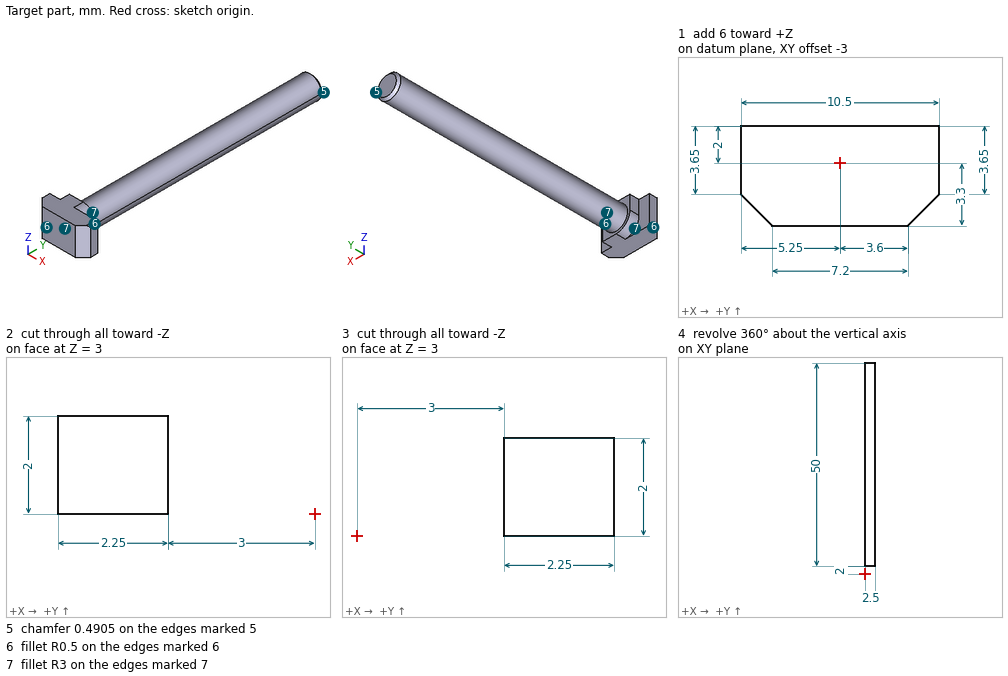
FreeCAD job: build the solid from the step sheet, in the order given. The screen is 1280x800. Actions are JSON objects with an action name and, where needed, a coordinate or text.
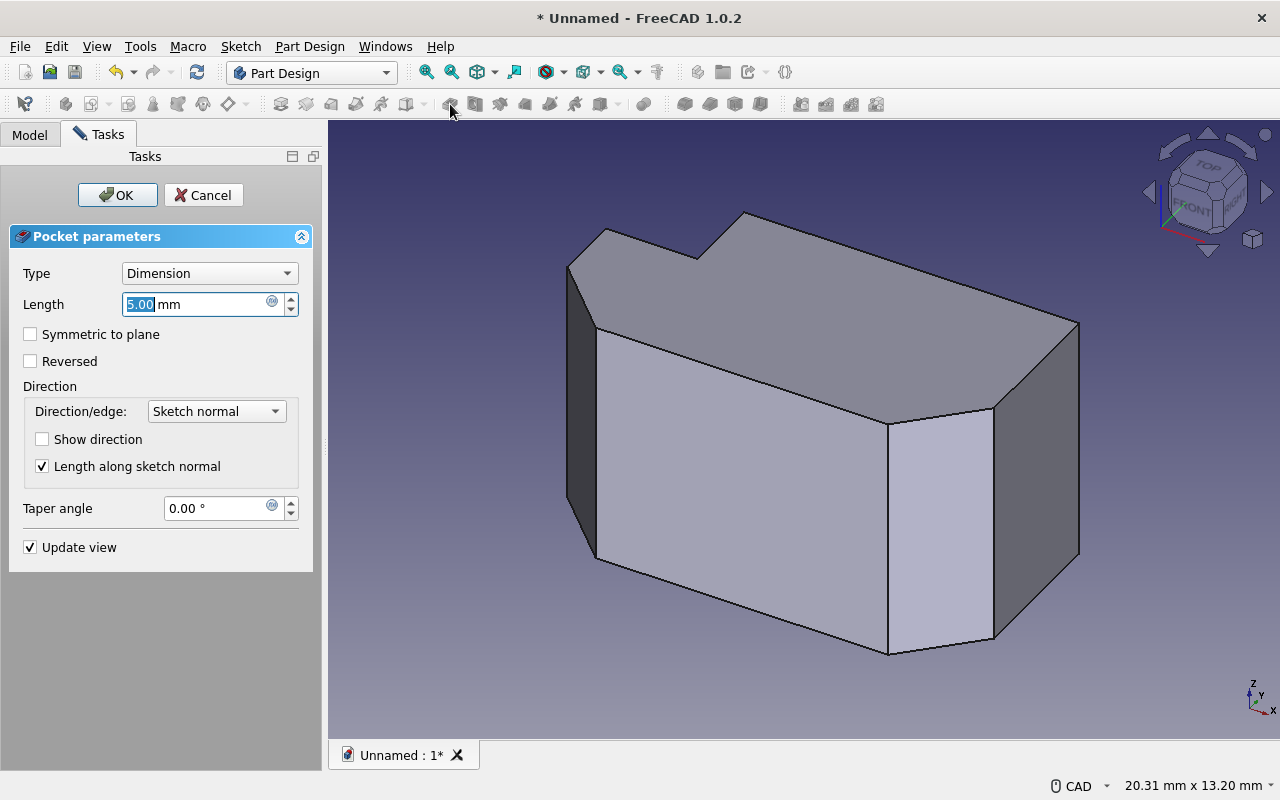
{"action": "left_click", "coordinate": [210, 274]}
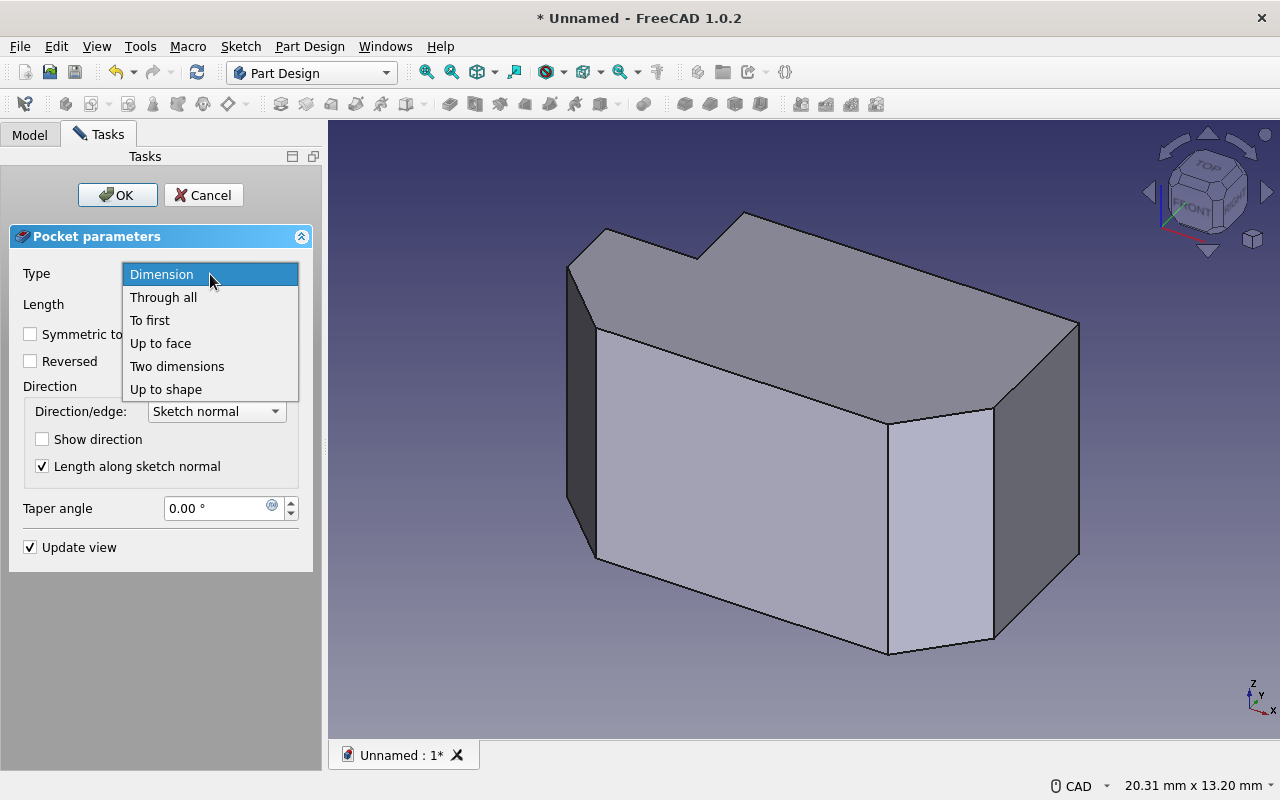
{"action": "left_click", "coordinate": [208, 298]}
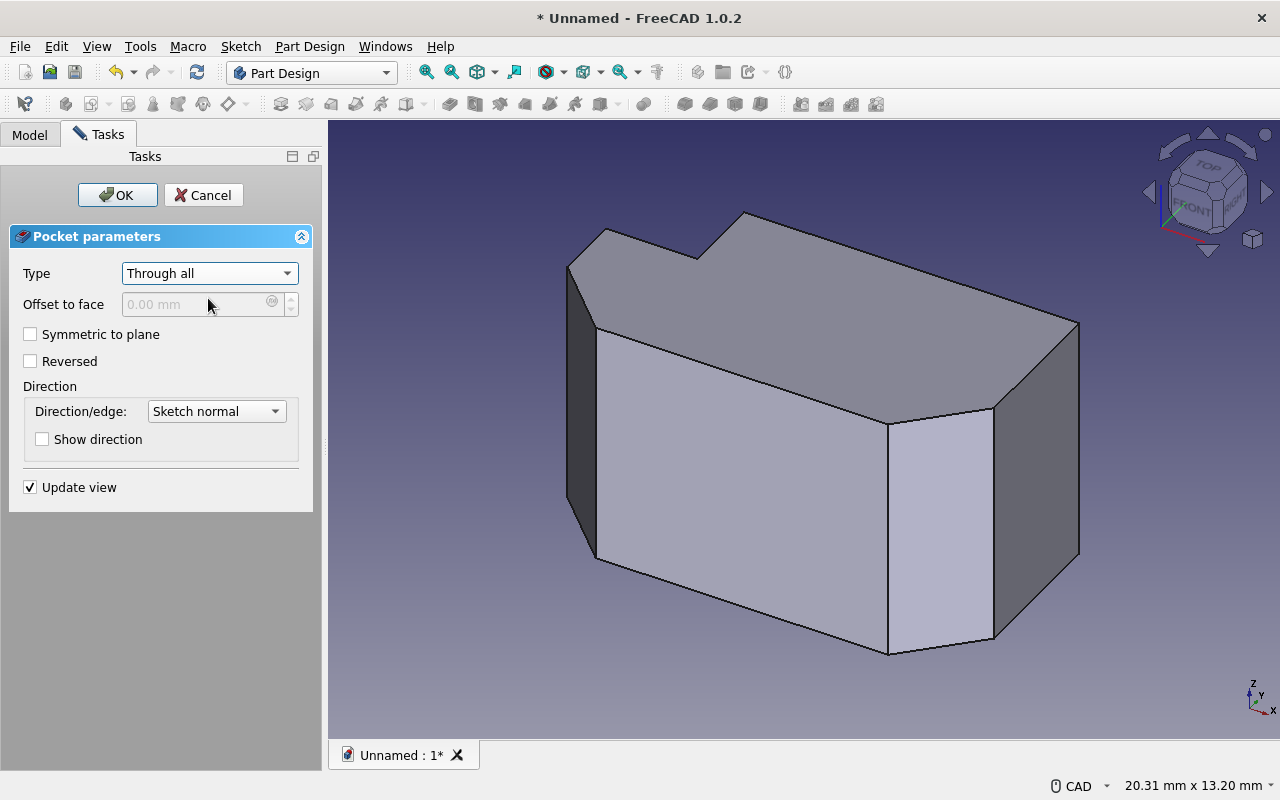
{"action": "left_click", "coordinate": [118, 195]}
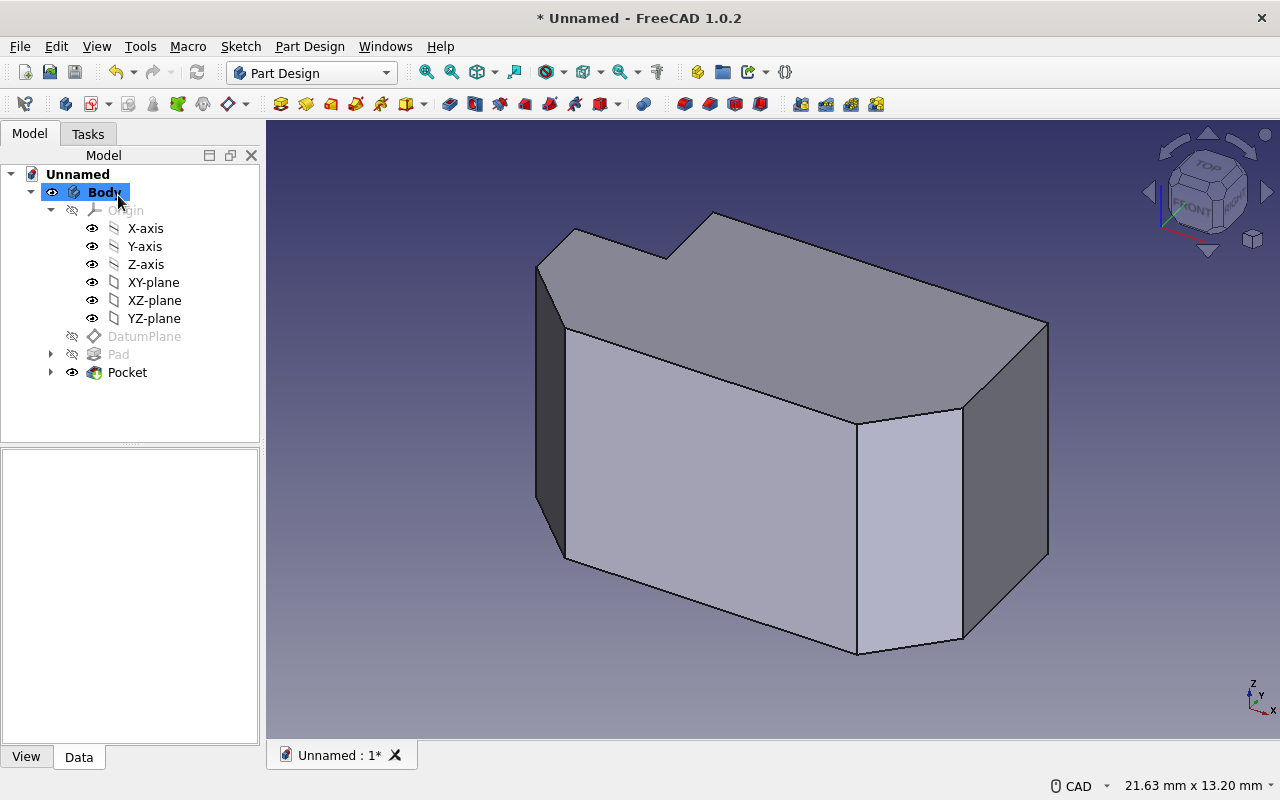
{"action": "left_click", "coordinate": [834, 333]}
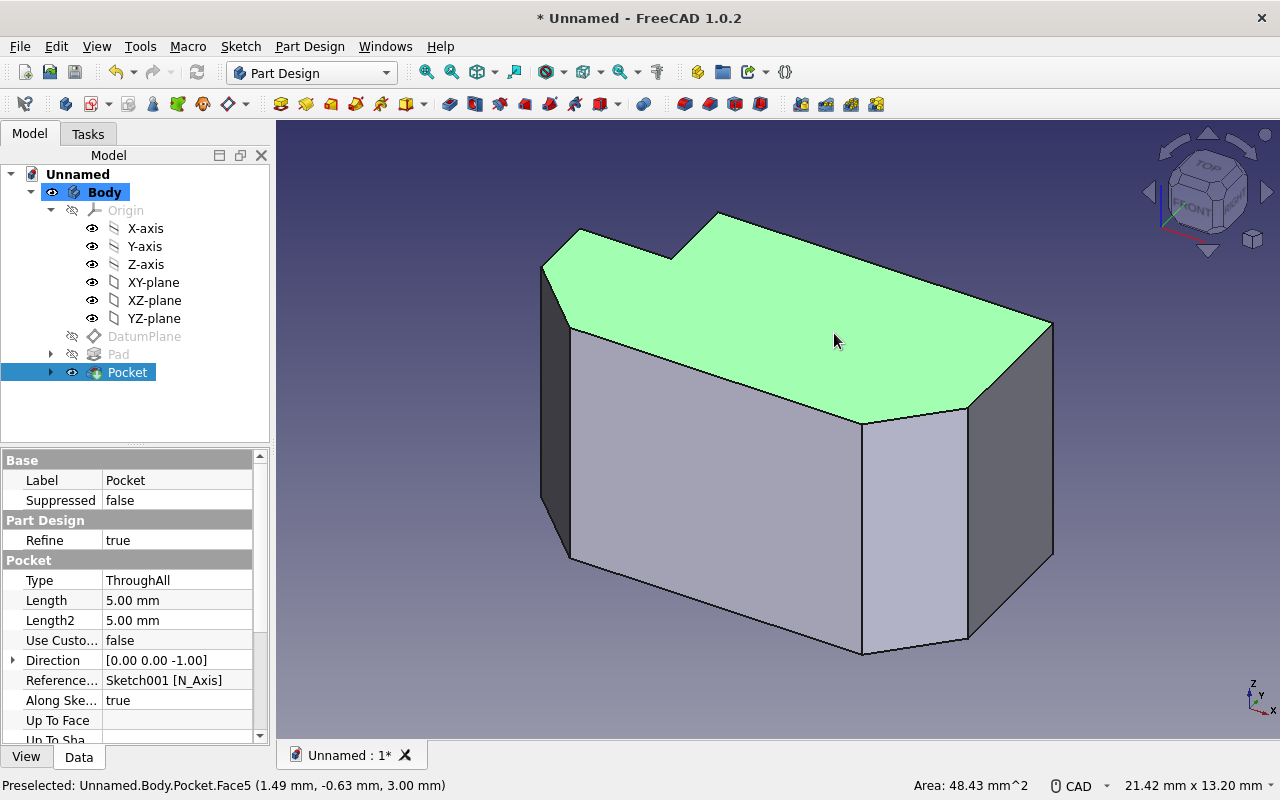
{"action": "left_click", "coordinate": [90, 104]}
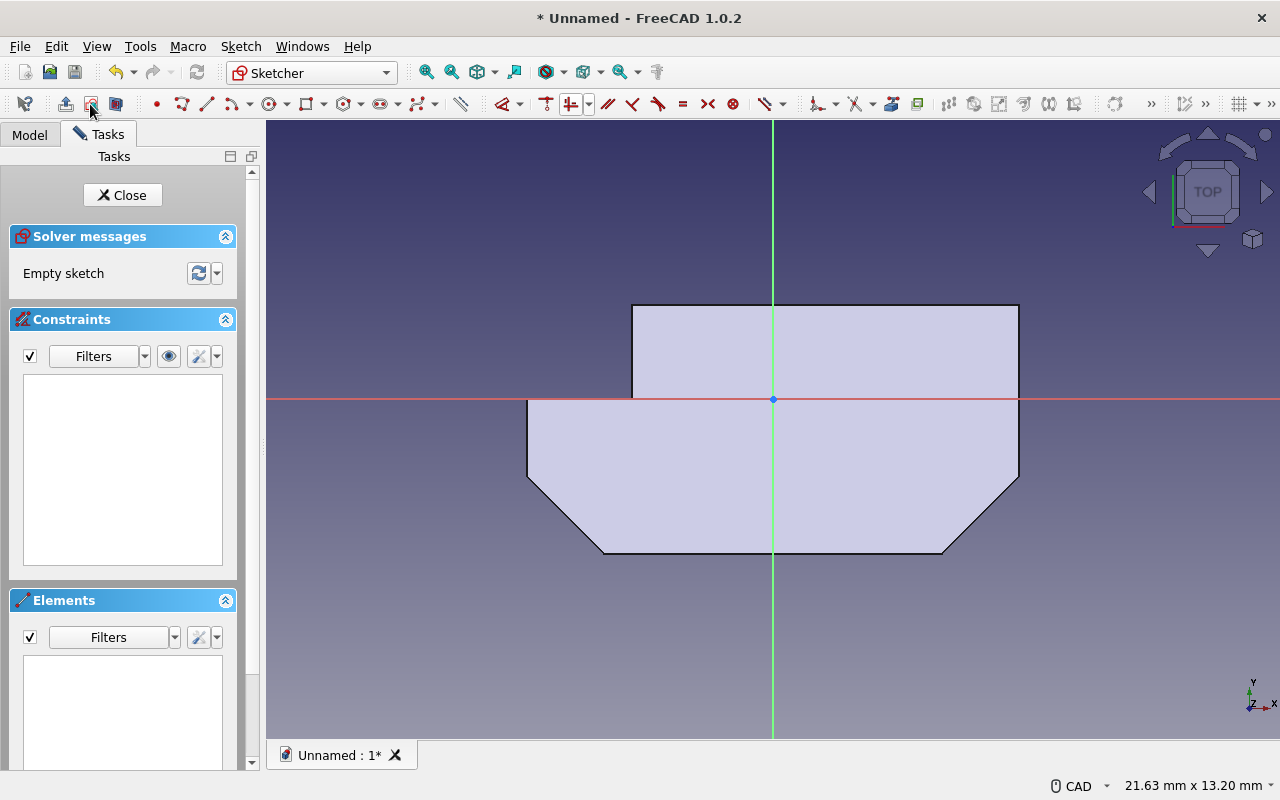
{"action": "scroll", "coordinate": [1052, 289], "scroll_direction": "up", "scroll_amount": 4}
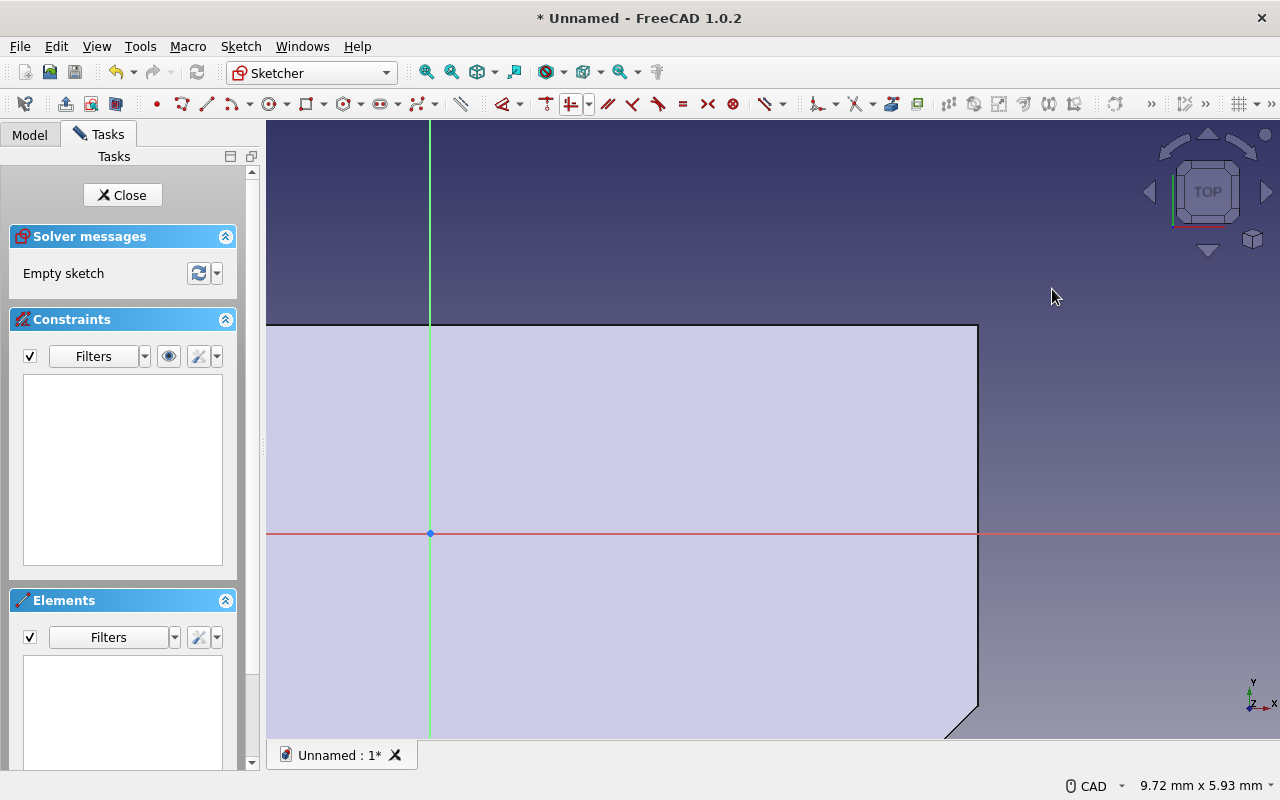
{"action": "left_click", "coordinate": [306, 104]}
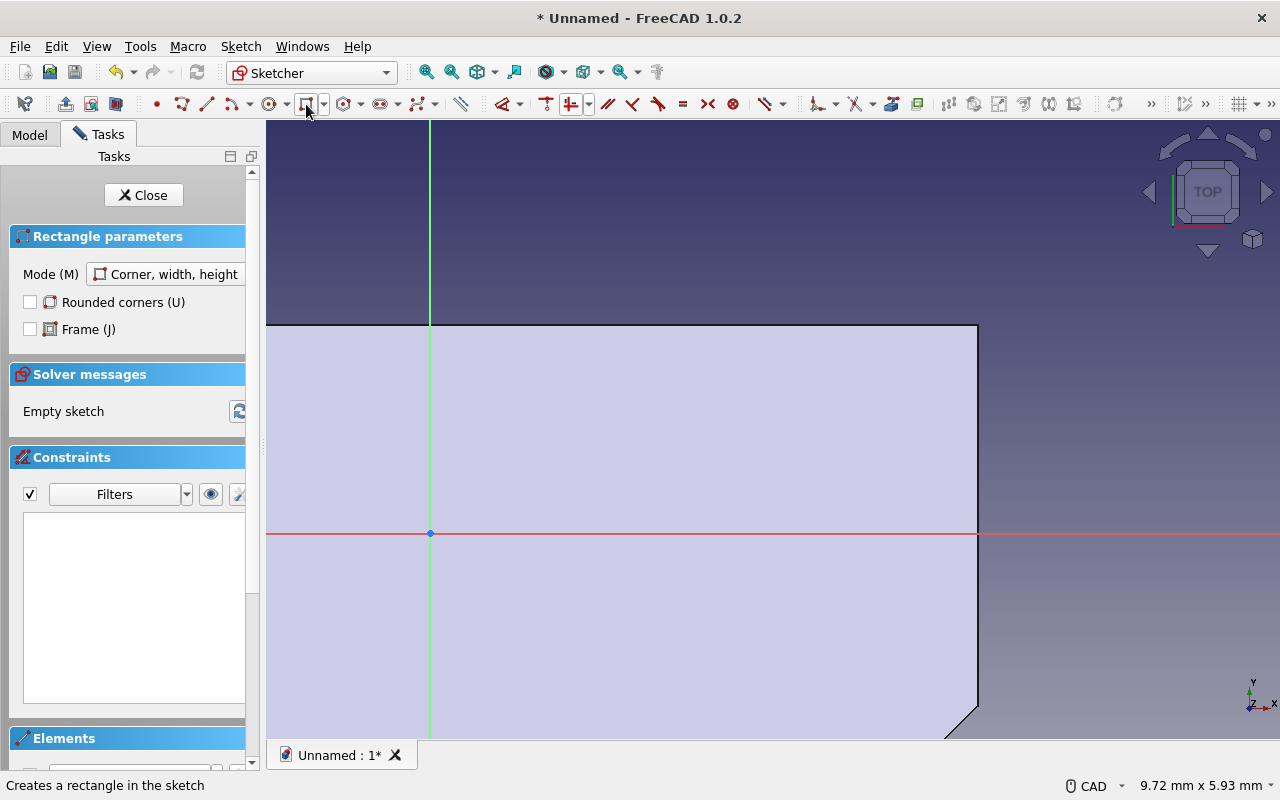
{"action": "left_click", "coordinate": [743, 325]}
{"action": "left_click", "coordinate": [978, 534]}
{"action": "key", "text": "Escape"}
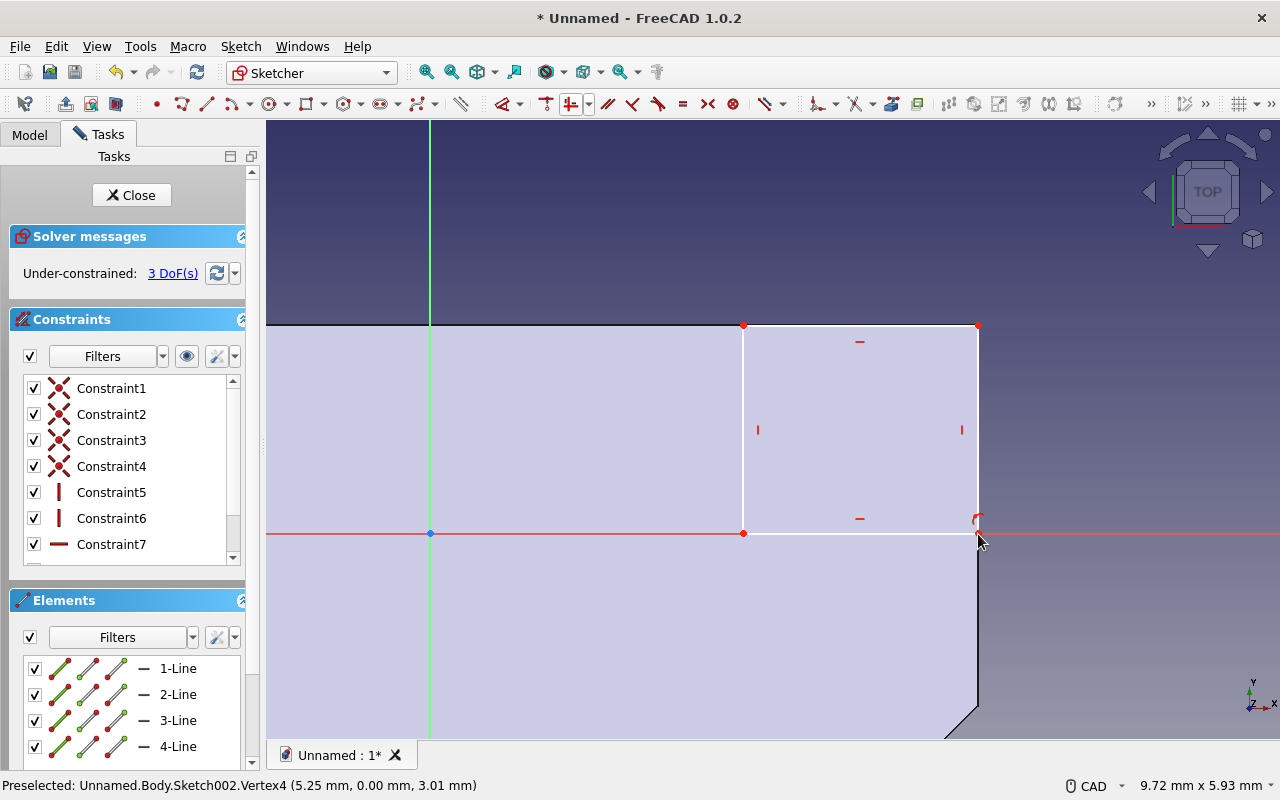
{"action": "key", "text": "d"}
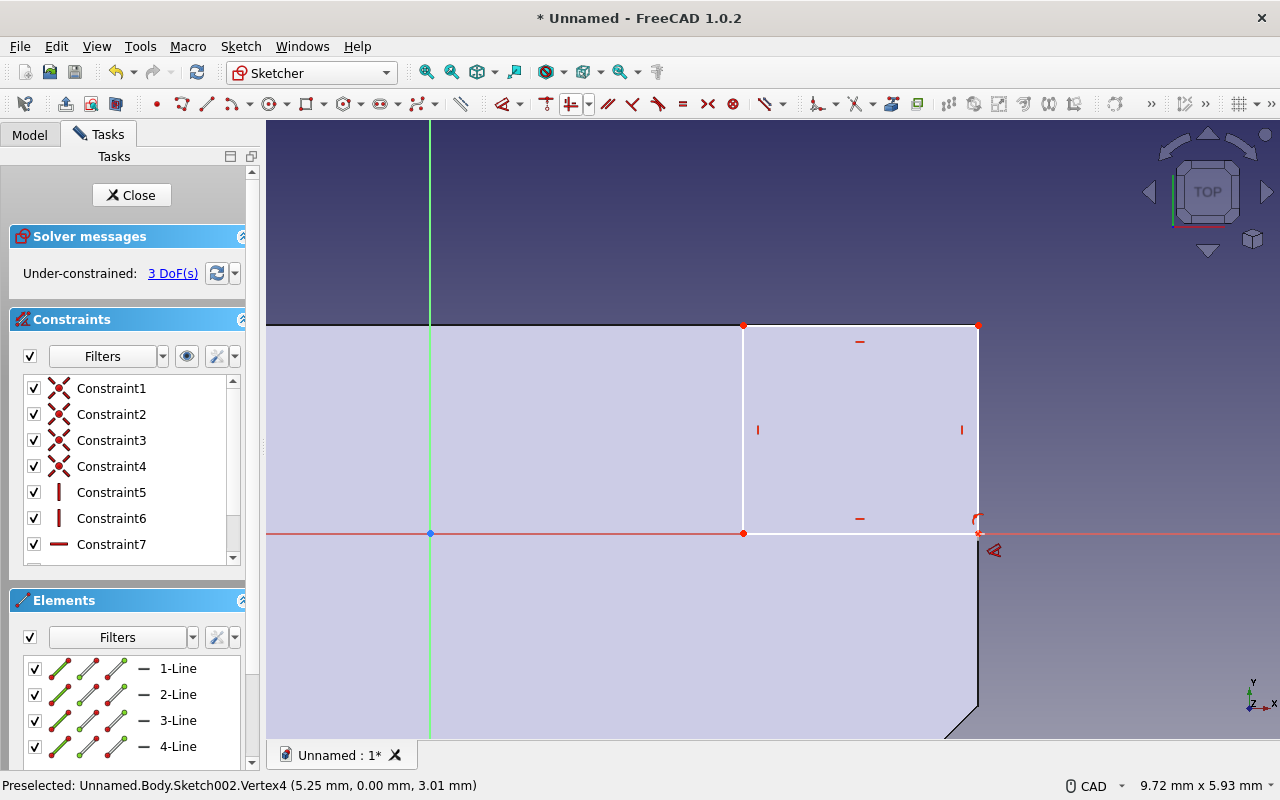
{"action": "left_click", "coordinate": [743, 388]}
{"action": "left_click", "coordinate": [777, 430]}